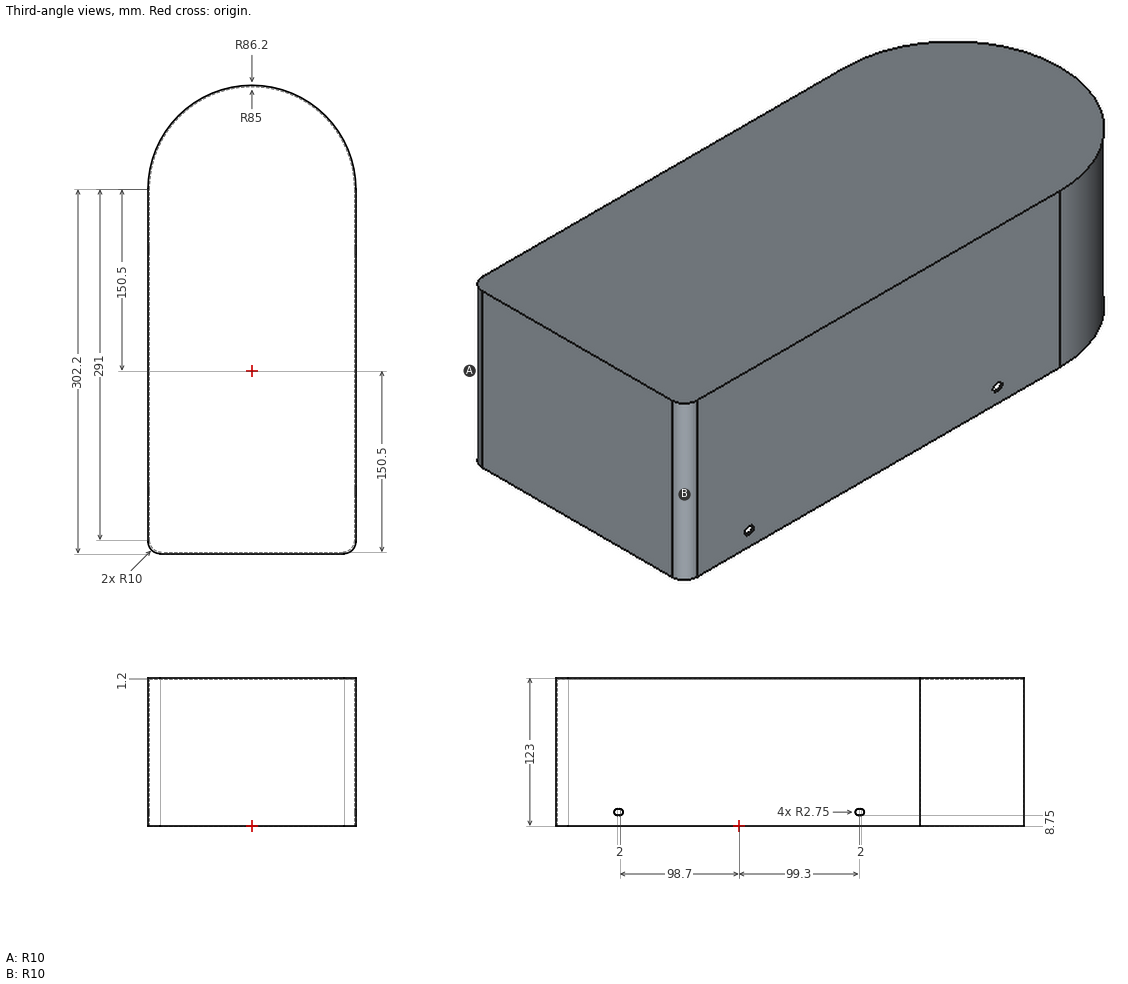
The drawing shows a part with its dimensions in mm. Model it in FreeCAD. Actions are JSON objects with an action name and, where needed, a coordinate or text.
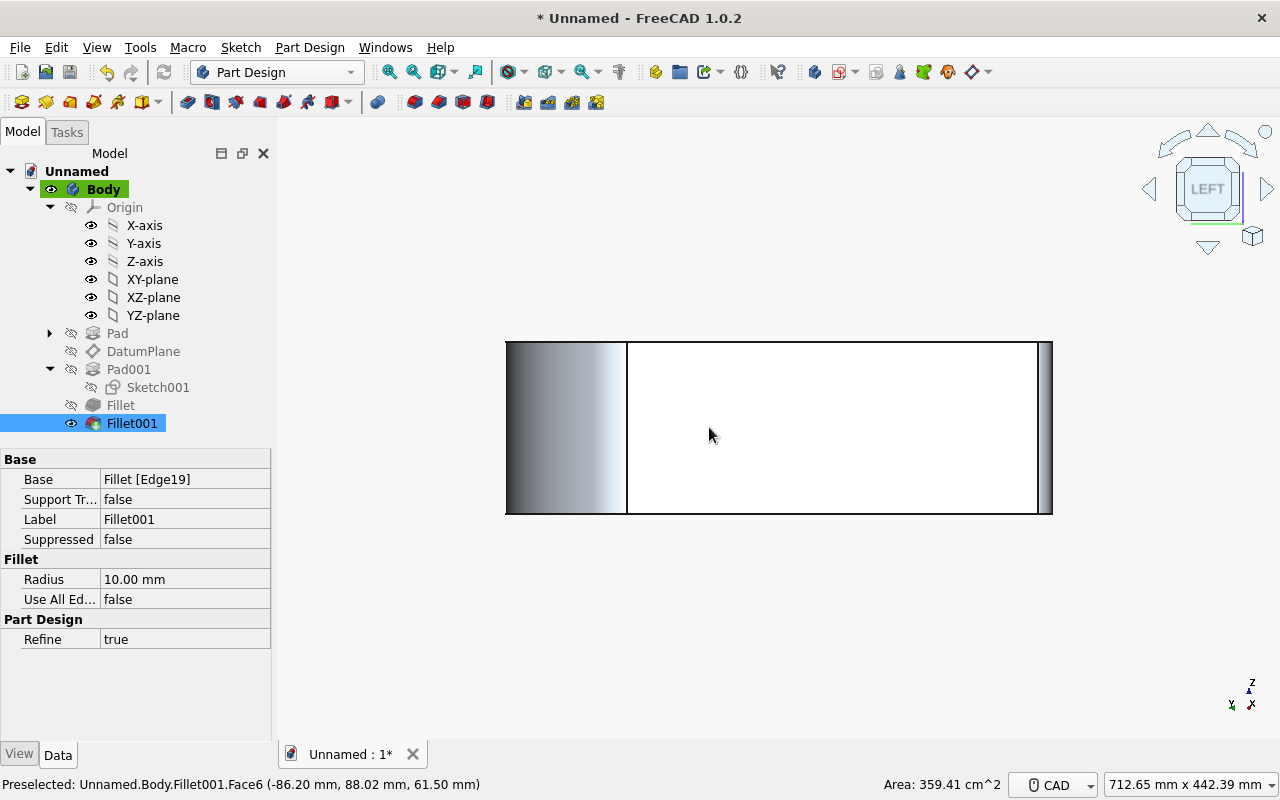
{"action": "left_click", "coordinate": [840, 72]}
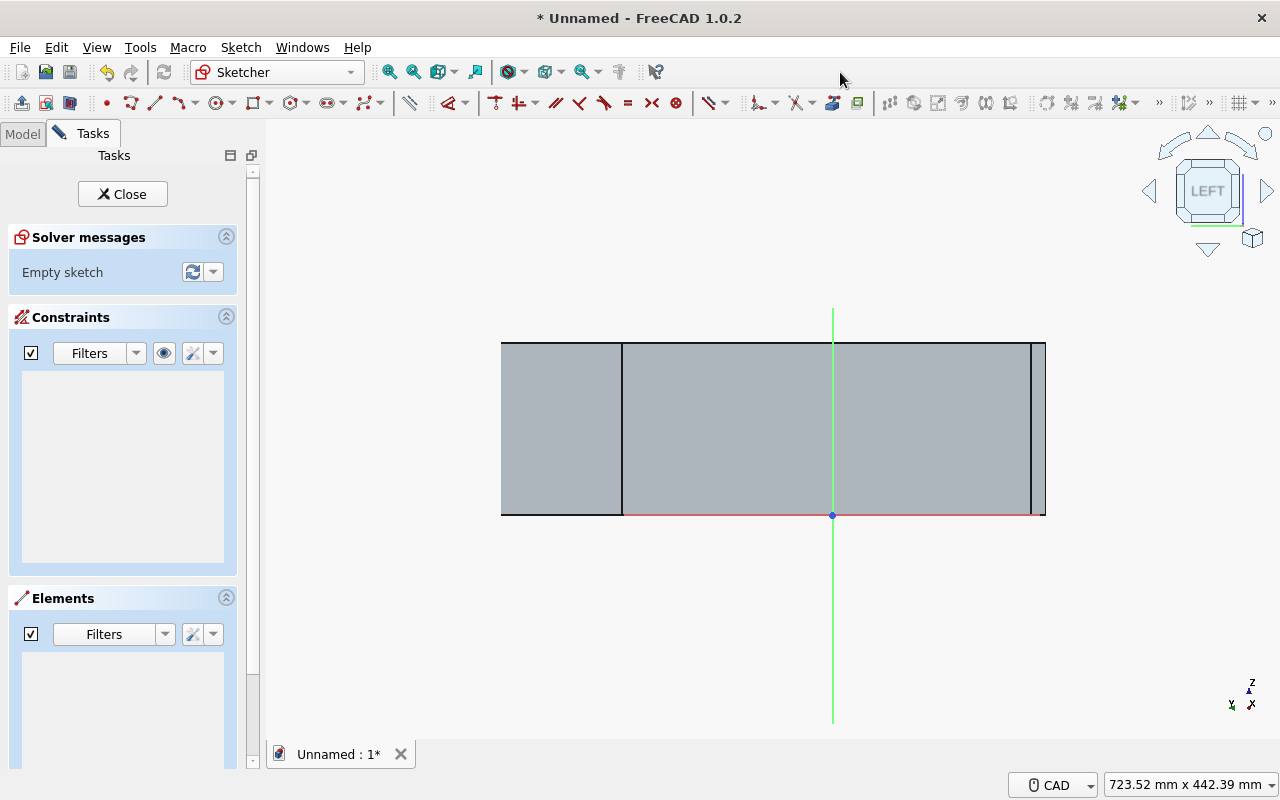
{"action": "scroll", "coordinate": [987, 598], "scroll_direction": "up", "scroll_amount": 3}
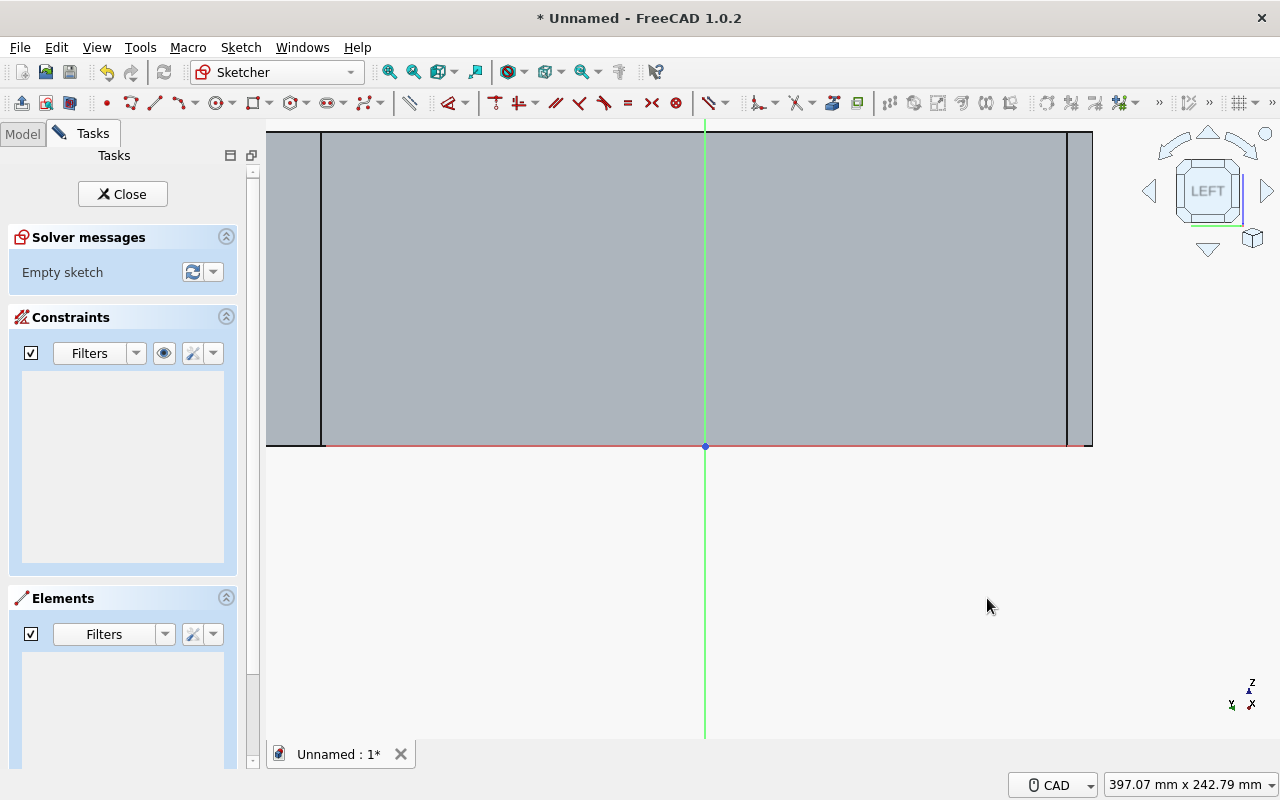
{"action": "left_click", "coordinate": [328, 104]}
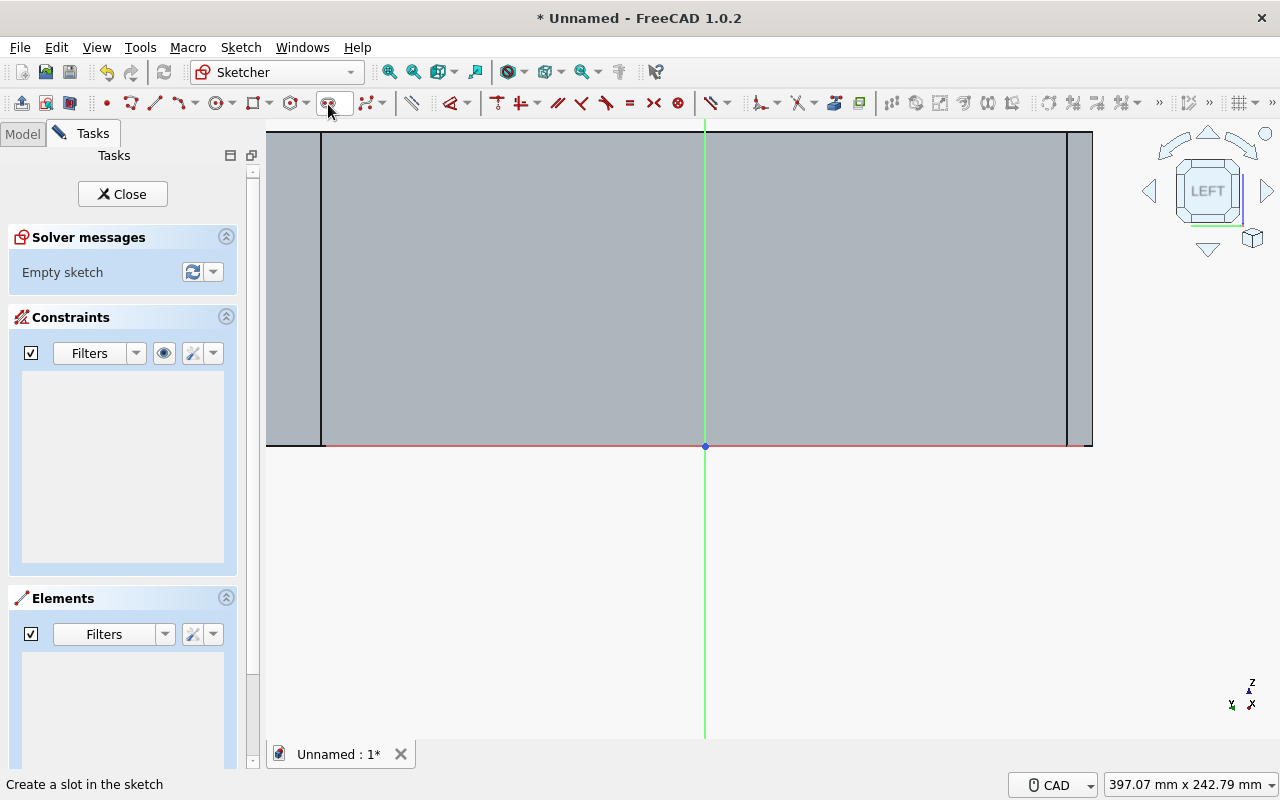
{"action": "scroll", "coordinate": [446, 417], "scroll_direction": "up", "scroll_amount": 6}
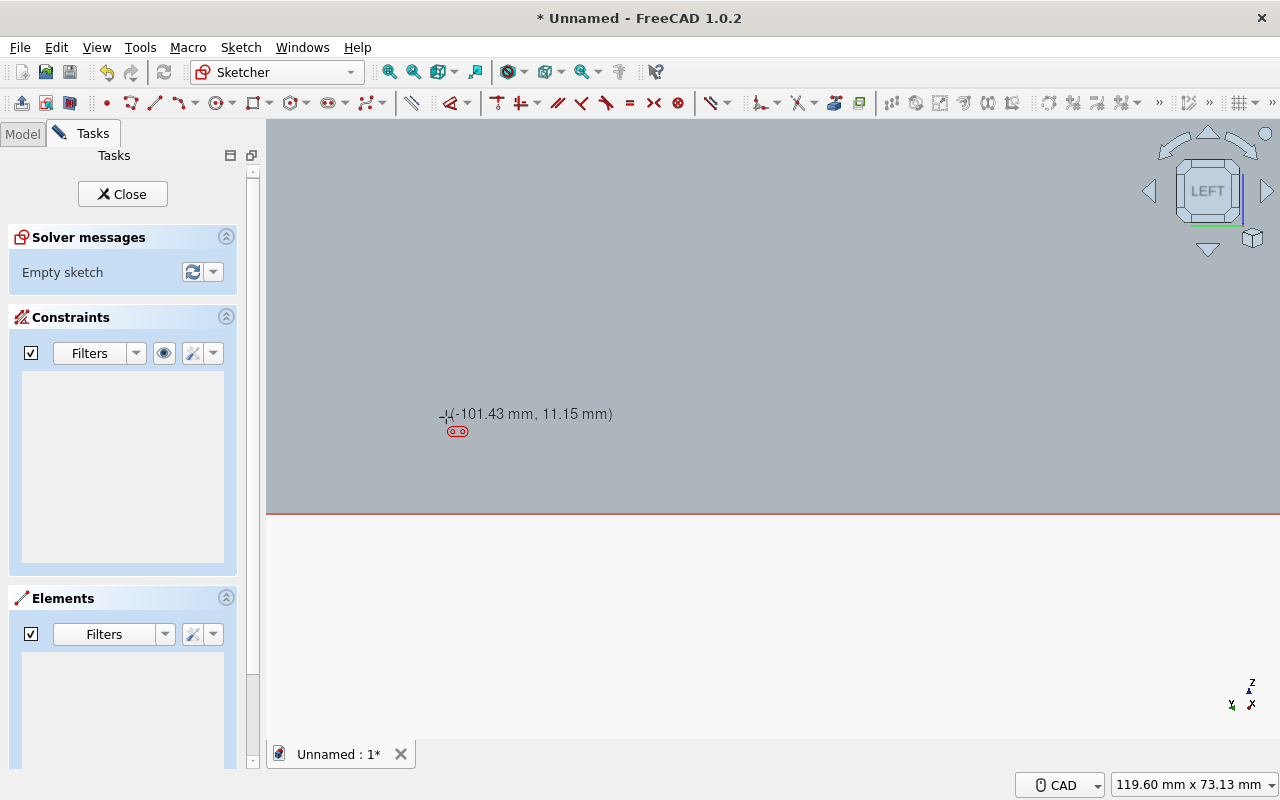
{"action": "left_click", "coordinate": [447, 416]}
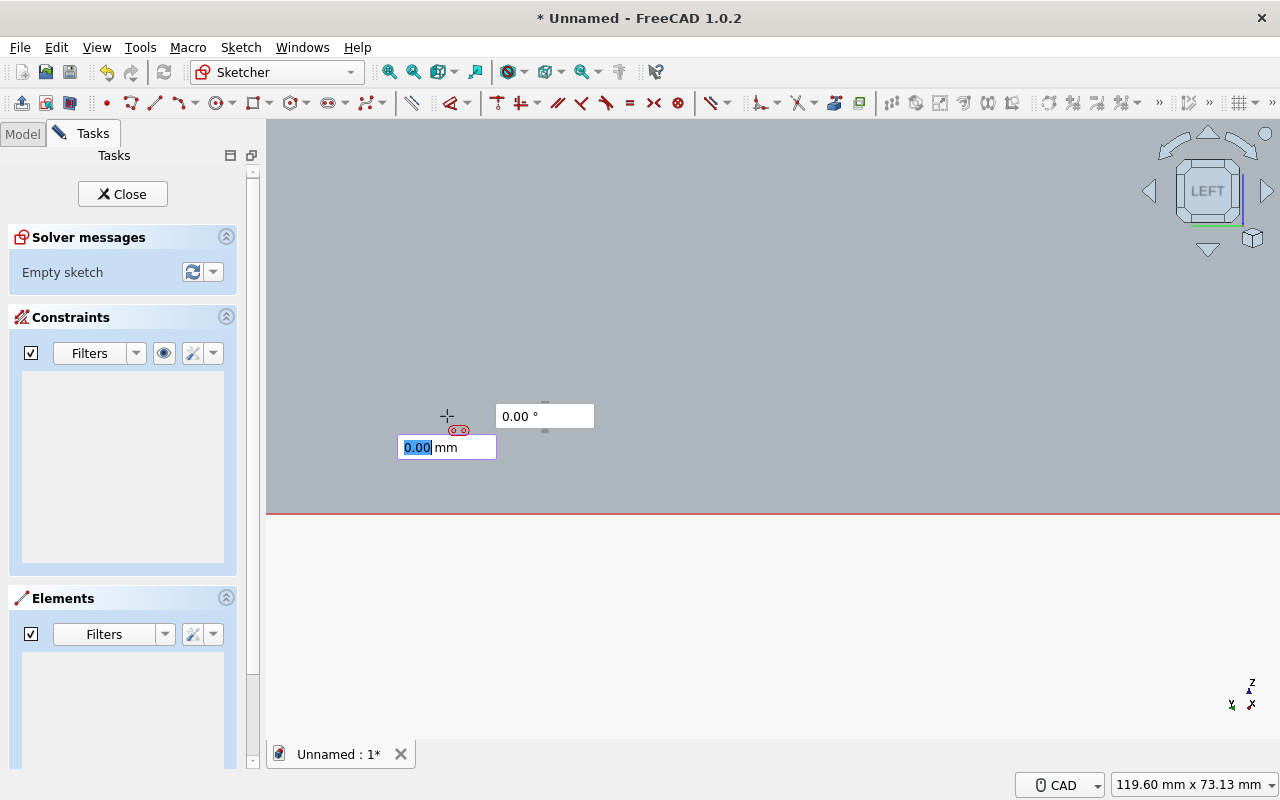
{"action": "left_click", "coordinate": [464, 416]}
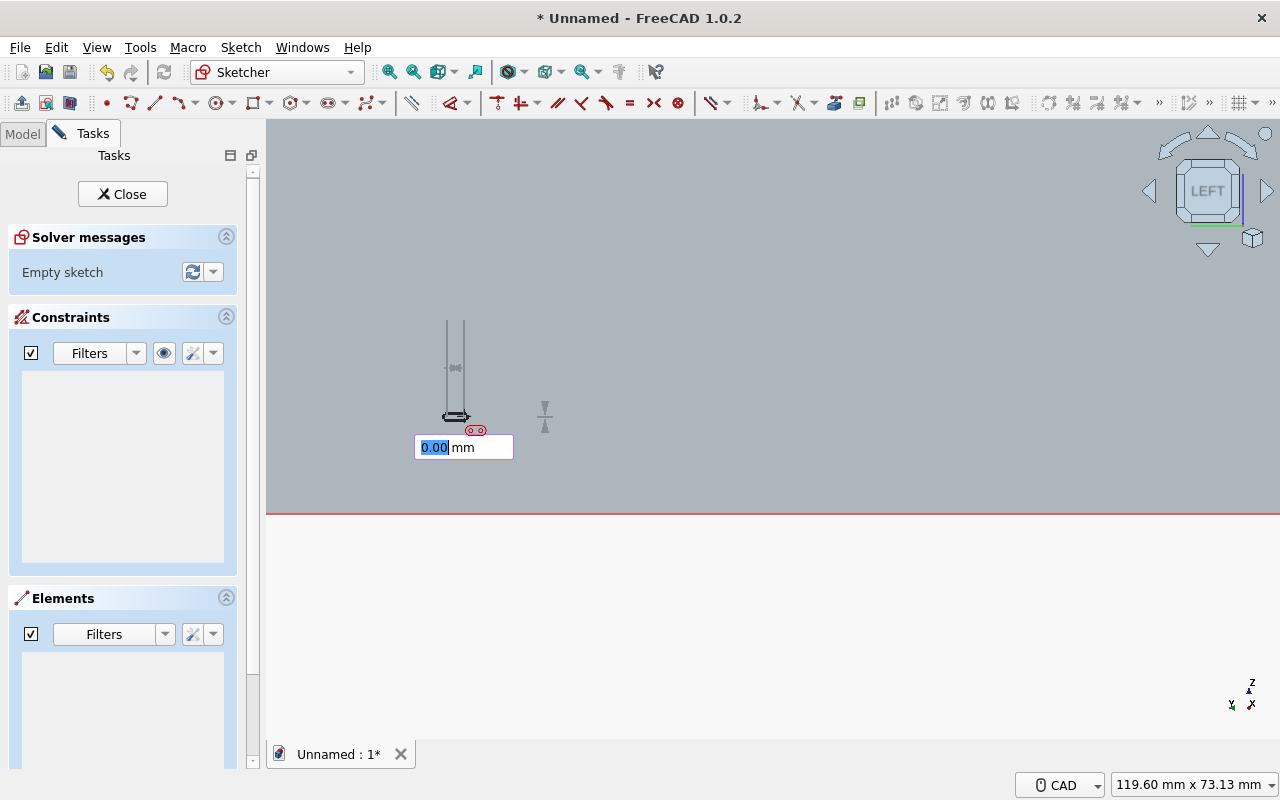
{"action": "left_click", "coordinate": [455, 440]}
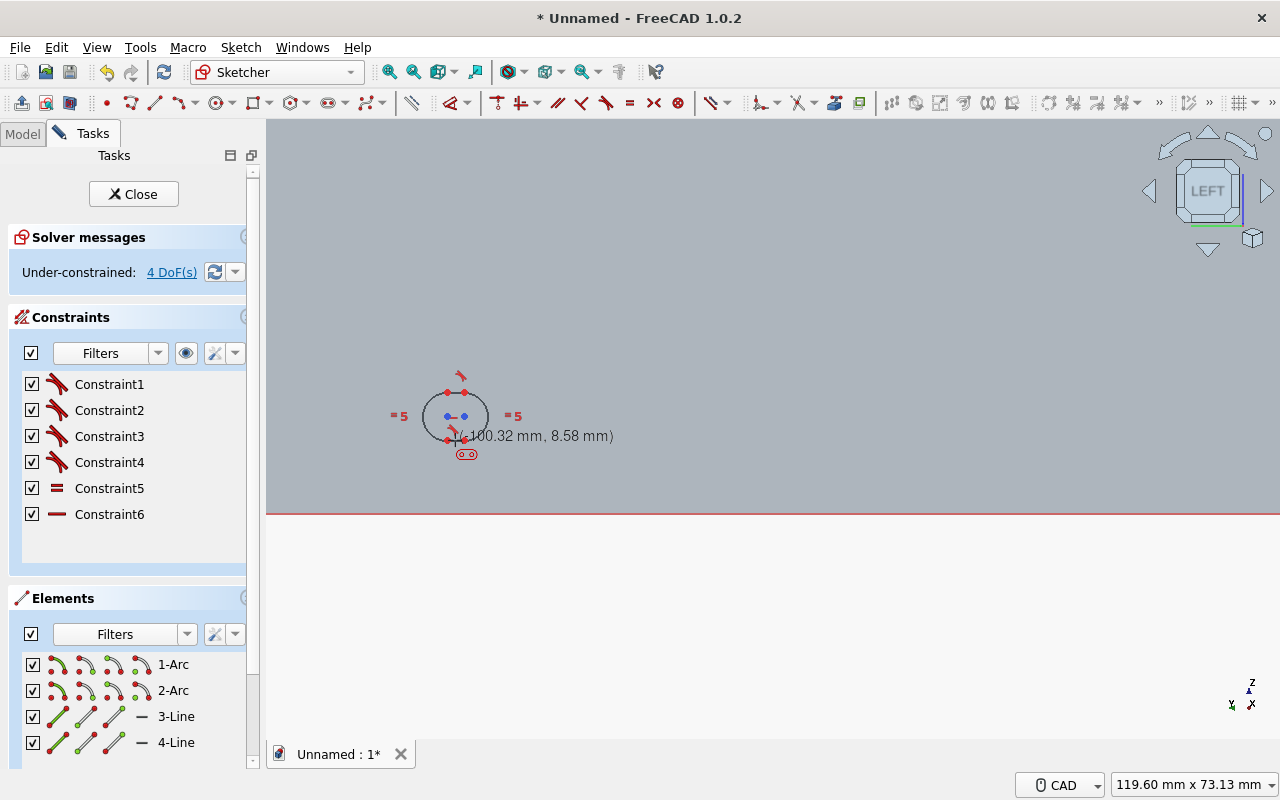
{"action": "scroll", "coordinate": [447, 419], "scroll_direction": "down", "scroll_amount": 6}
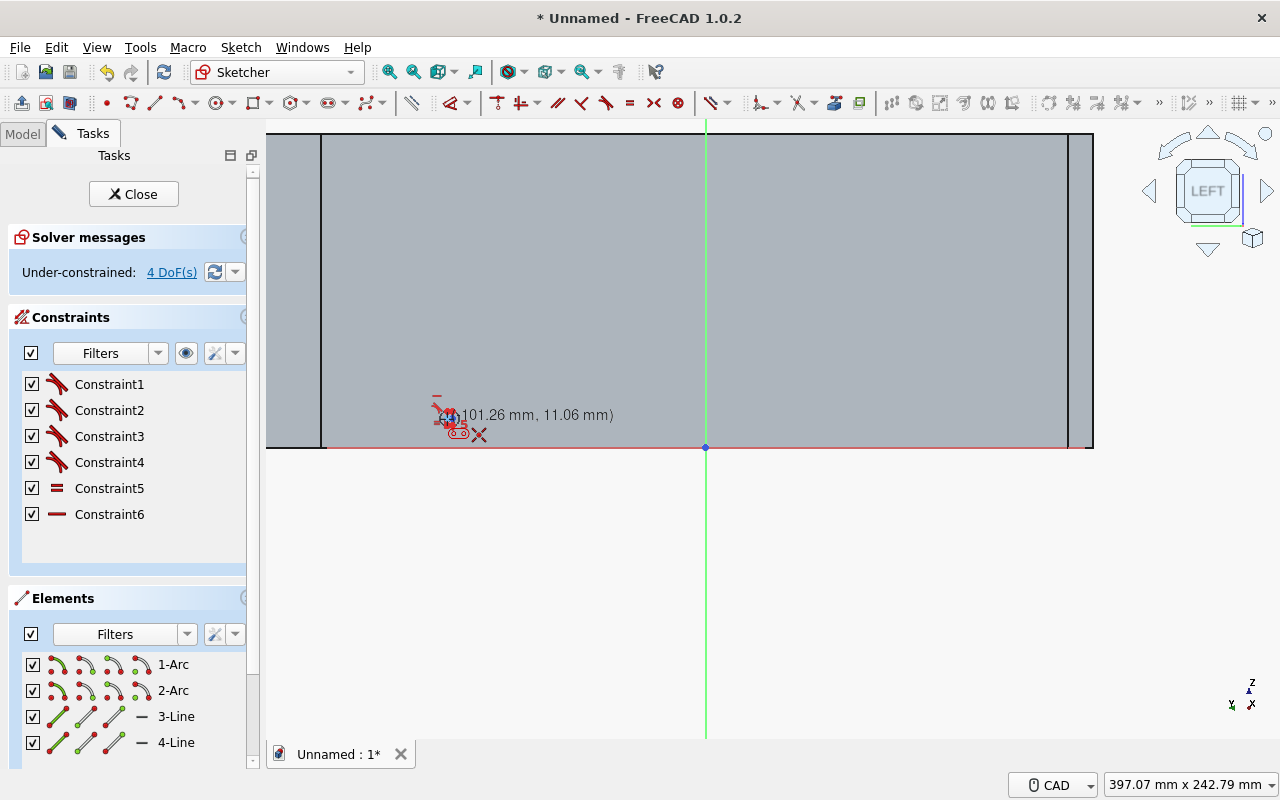
{"action": "scroll", "coordinate": [958, 419], "scroll_direction": "up", "scroll_amount": 6}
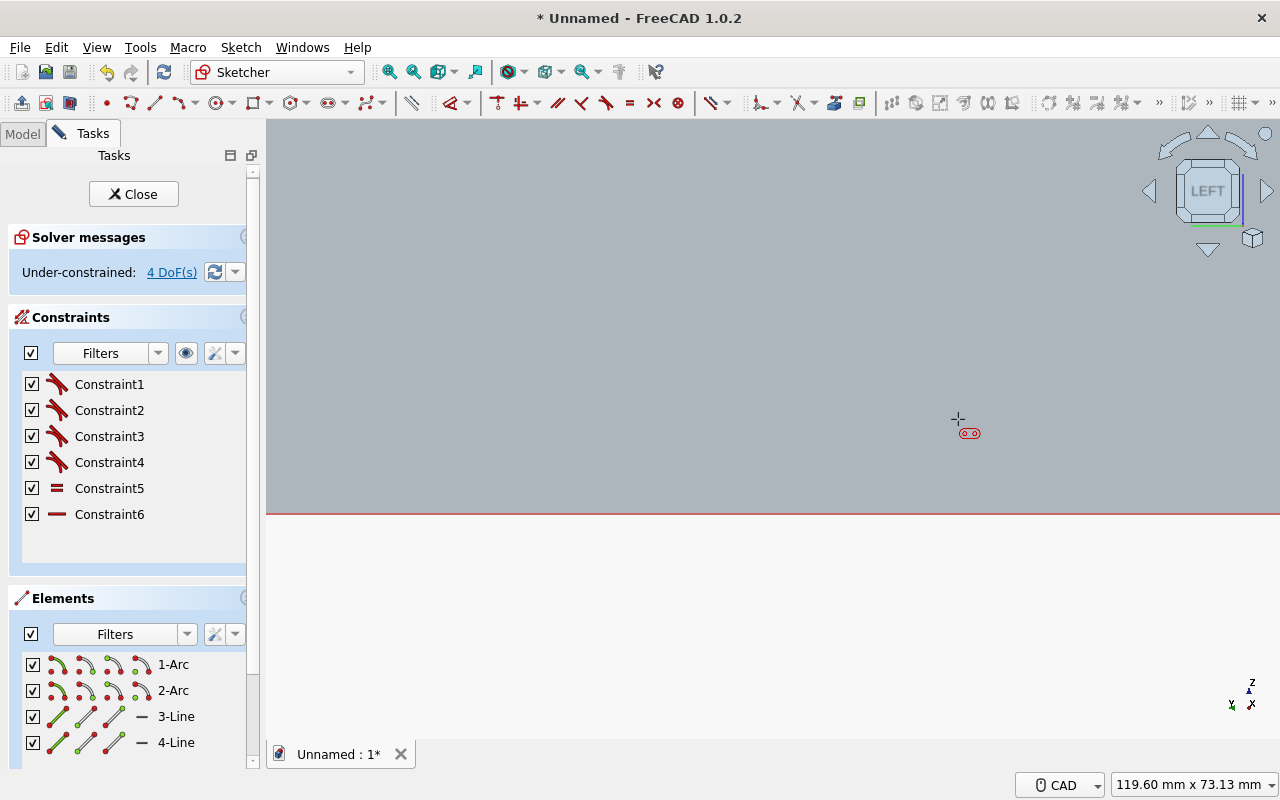
{"action": "left_click", "coordinate": [956, 416]}